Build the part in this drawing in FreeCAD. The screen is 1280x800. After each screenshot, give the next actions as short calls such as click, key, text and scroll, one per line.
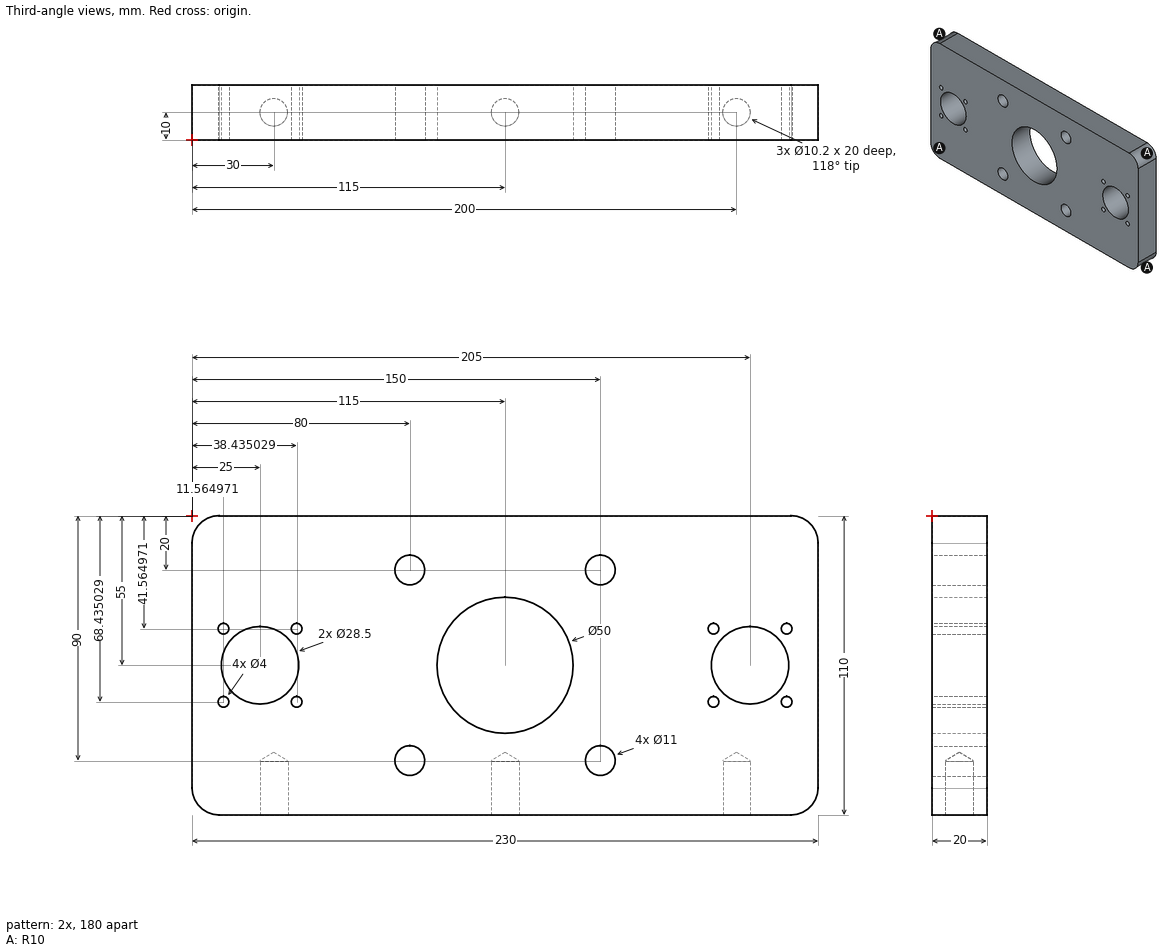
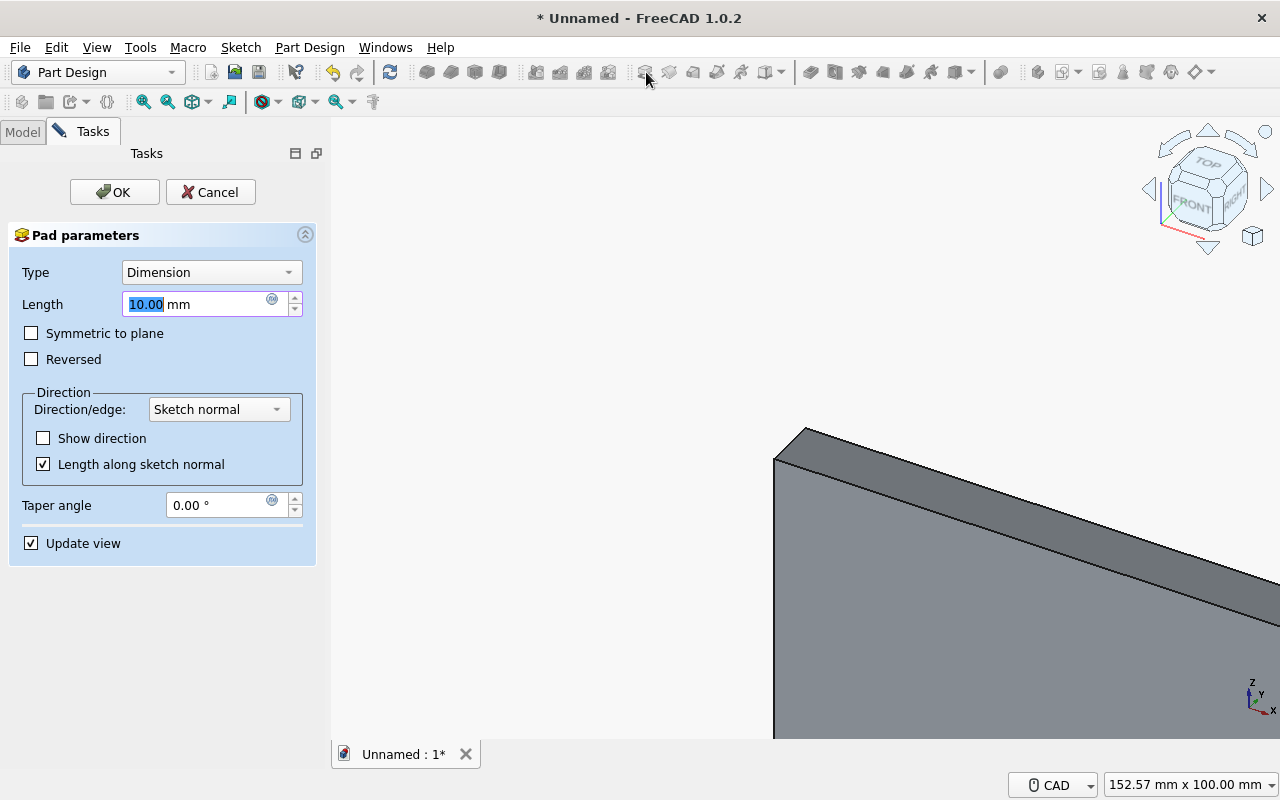
text(20)
key(Tab)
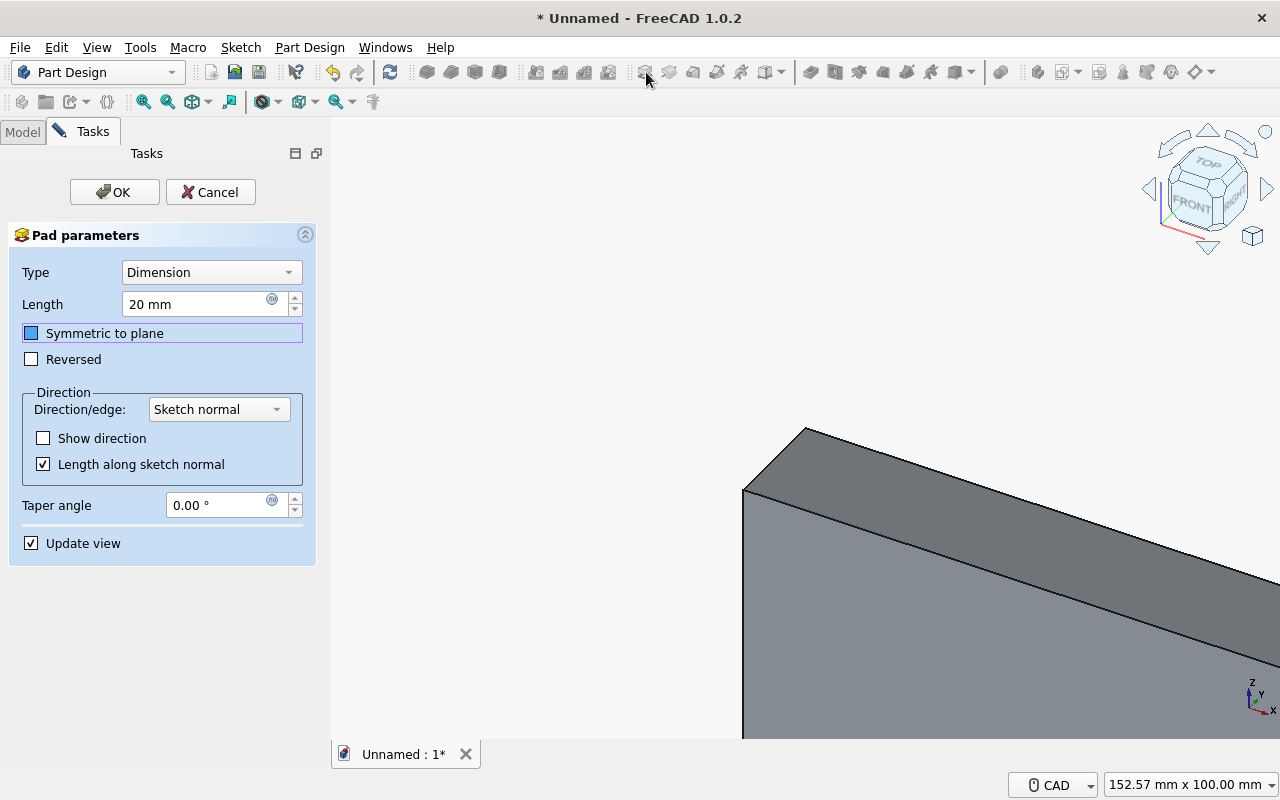
click(30, 359)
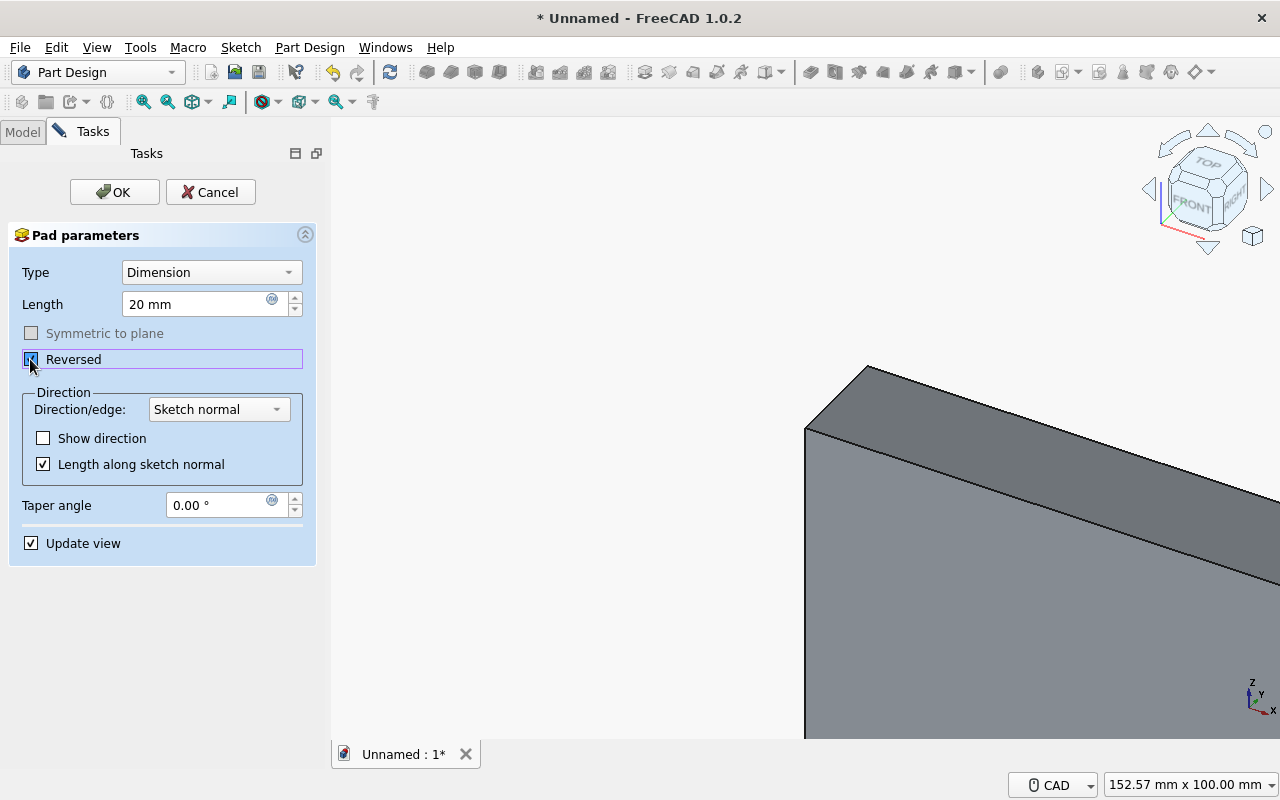
click(115, 192)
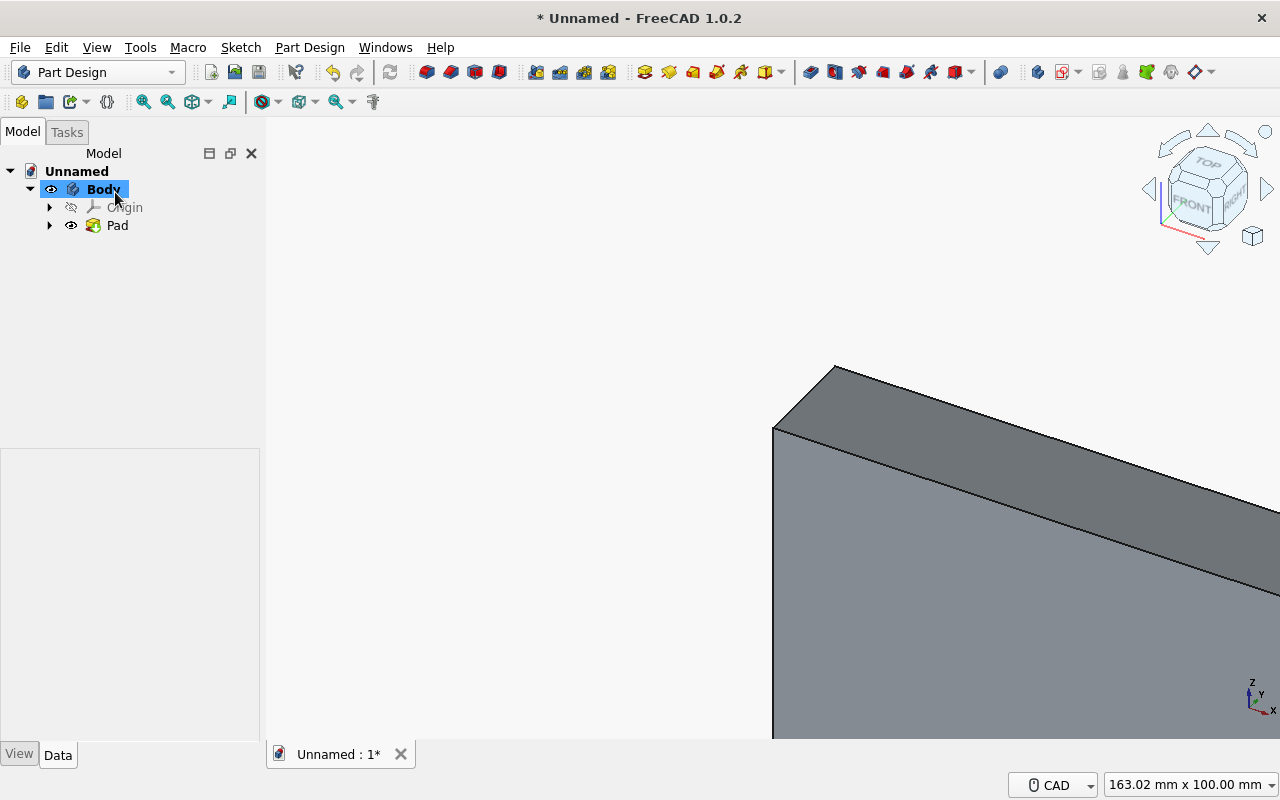
key(v)
key(f)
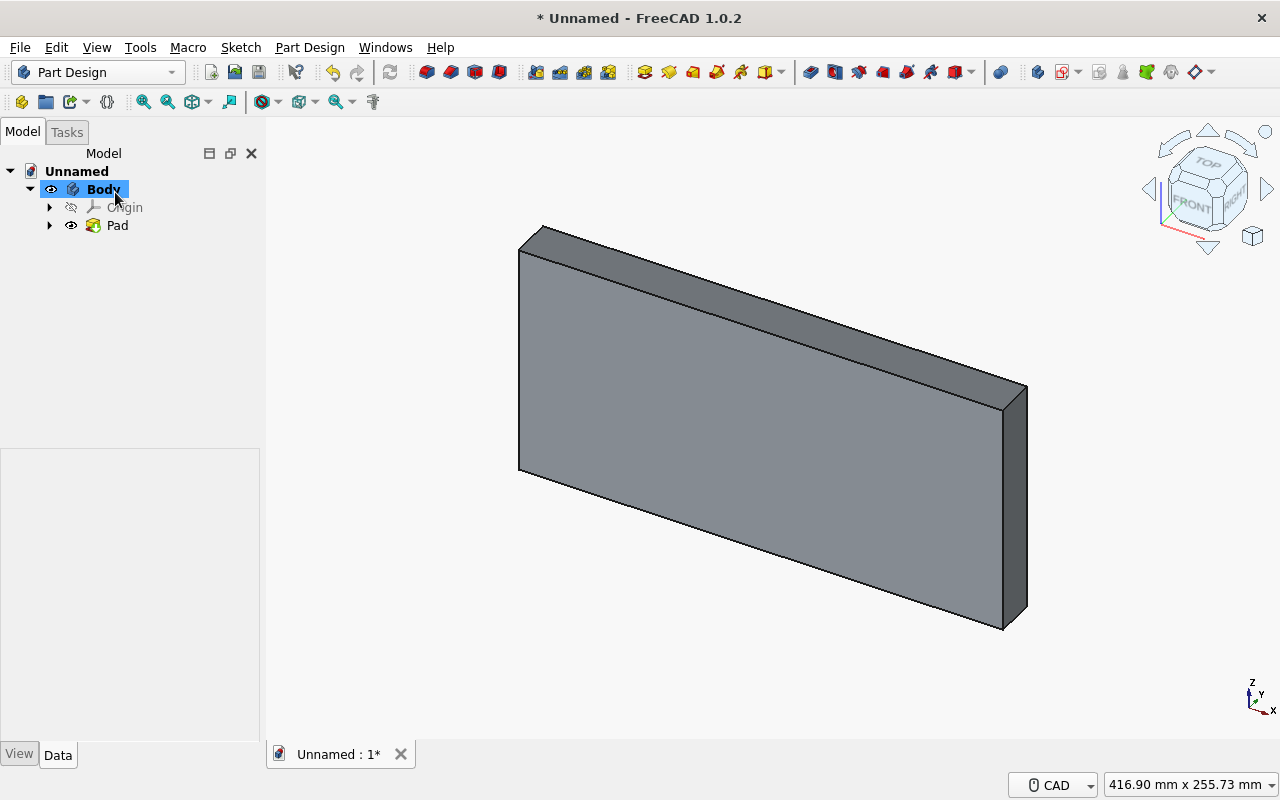
key(4)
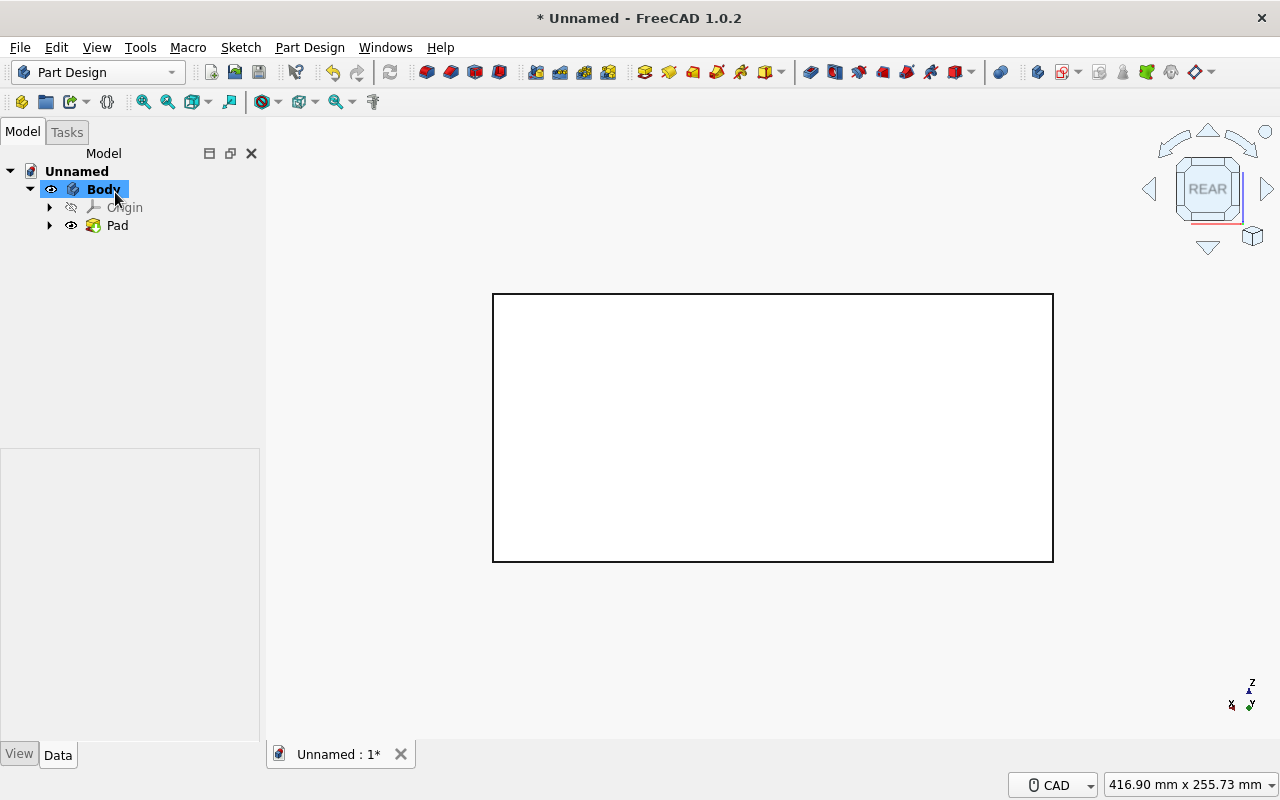
click(693, 427)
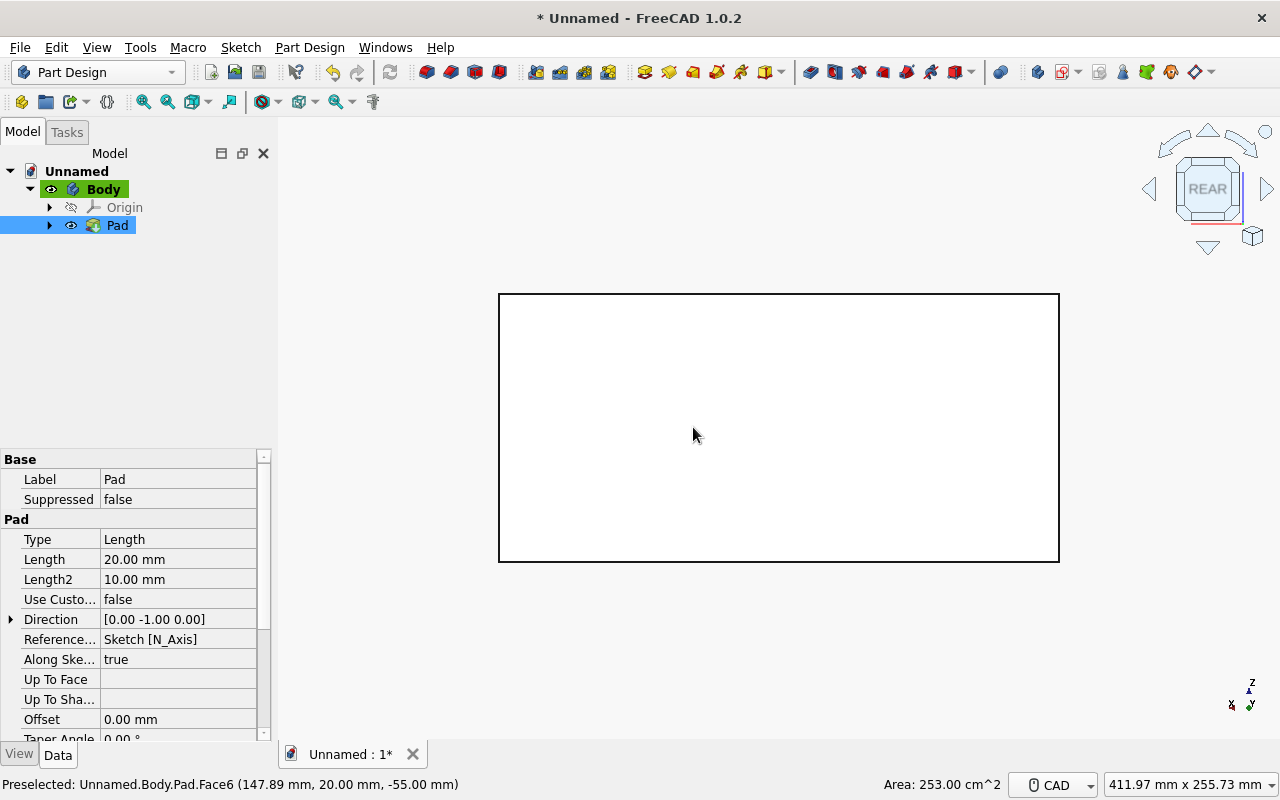
click(1062, 72)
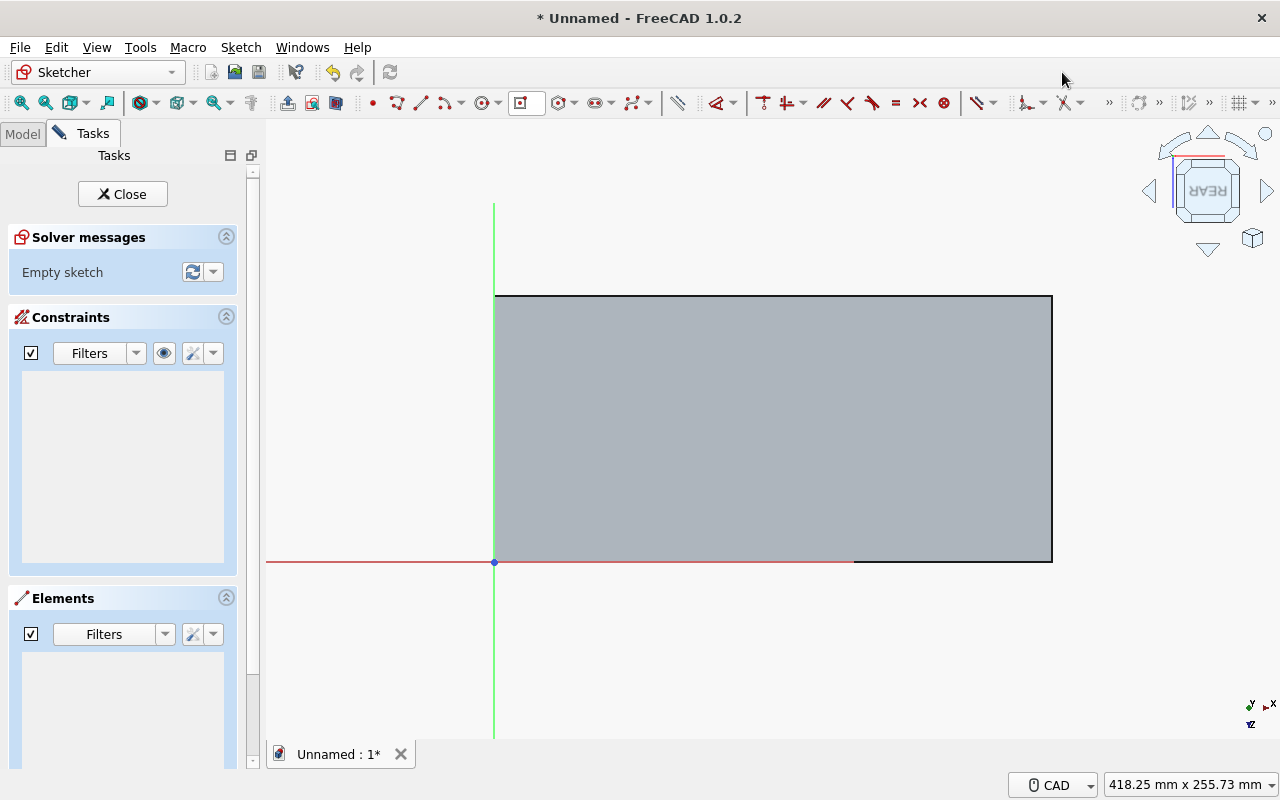
key(g)
key(c)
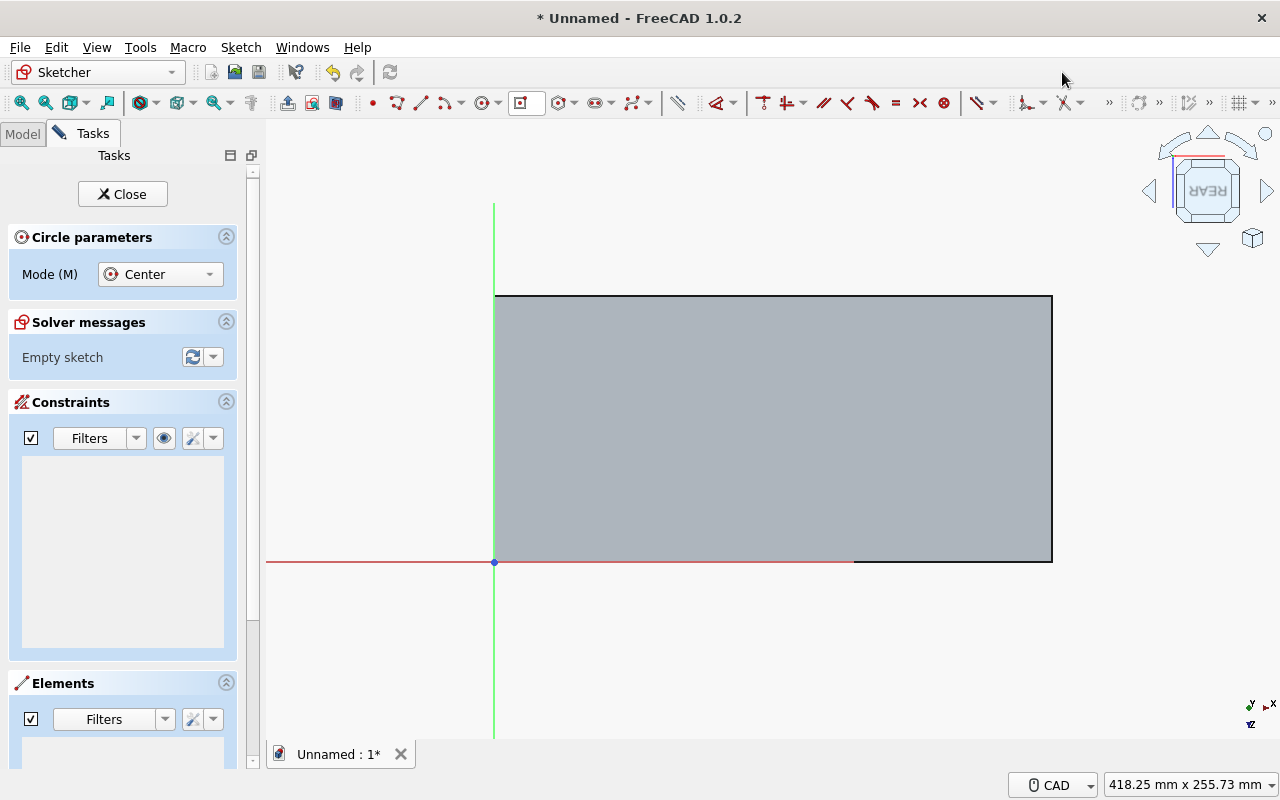
click(555, 429)
move(579, 405)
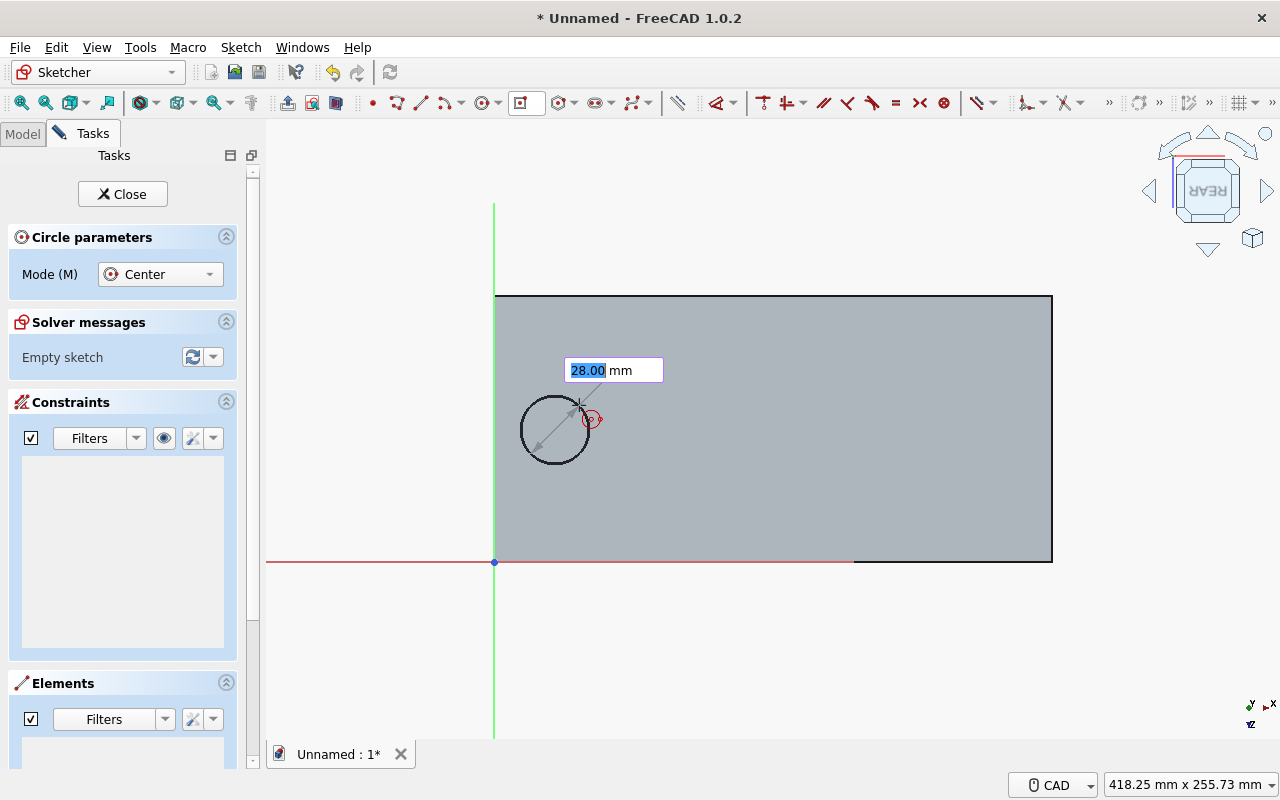
text(28.5)
key(Return)